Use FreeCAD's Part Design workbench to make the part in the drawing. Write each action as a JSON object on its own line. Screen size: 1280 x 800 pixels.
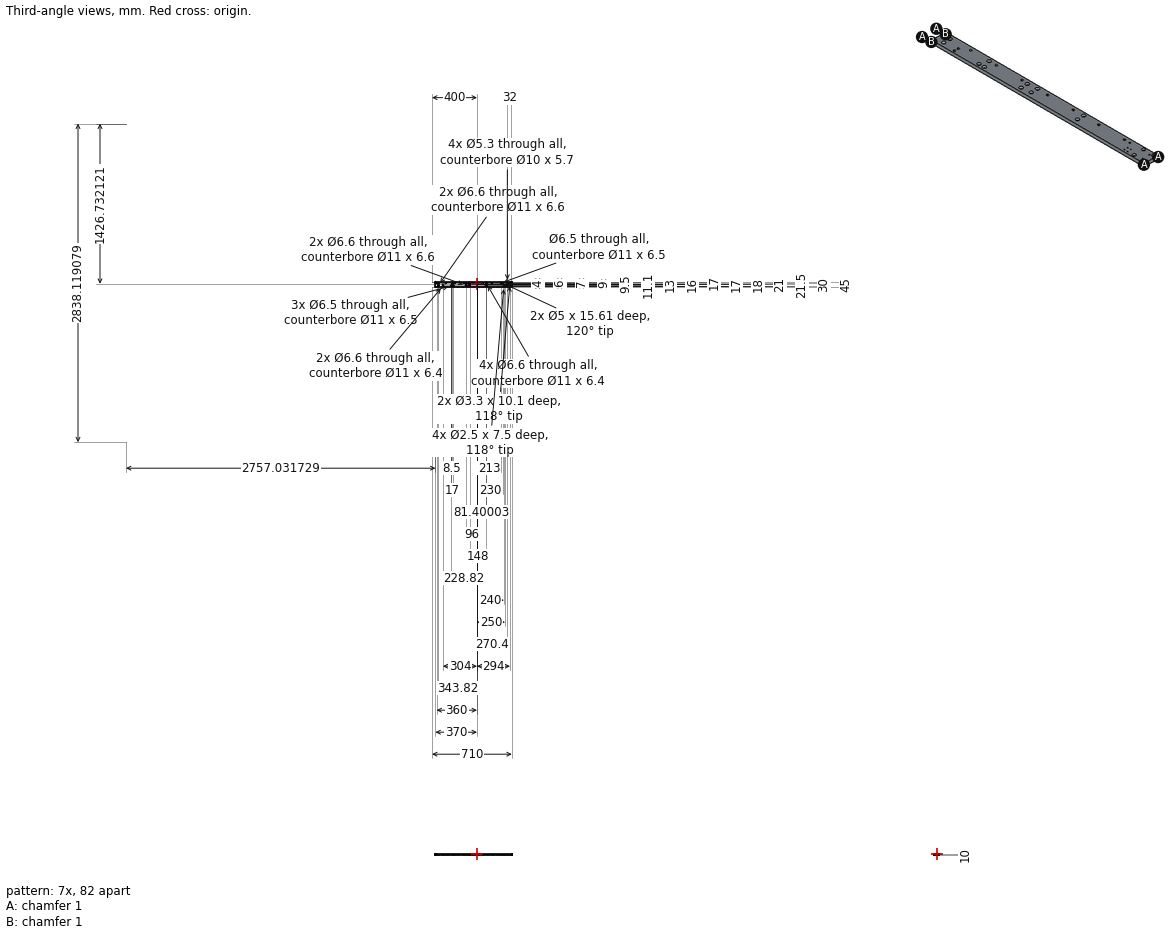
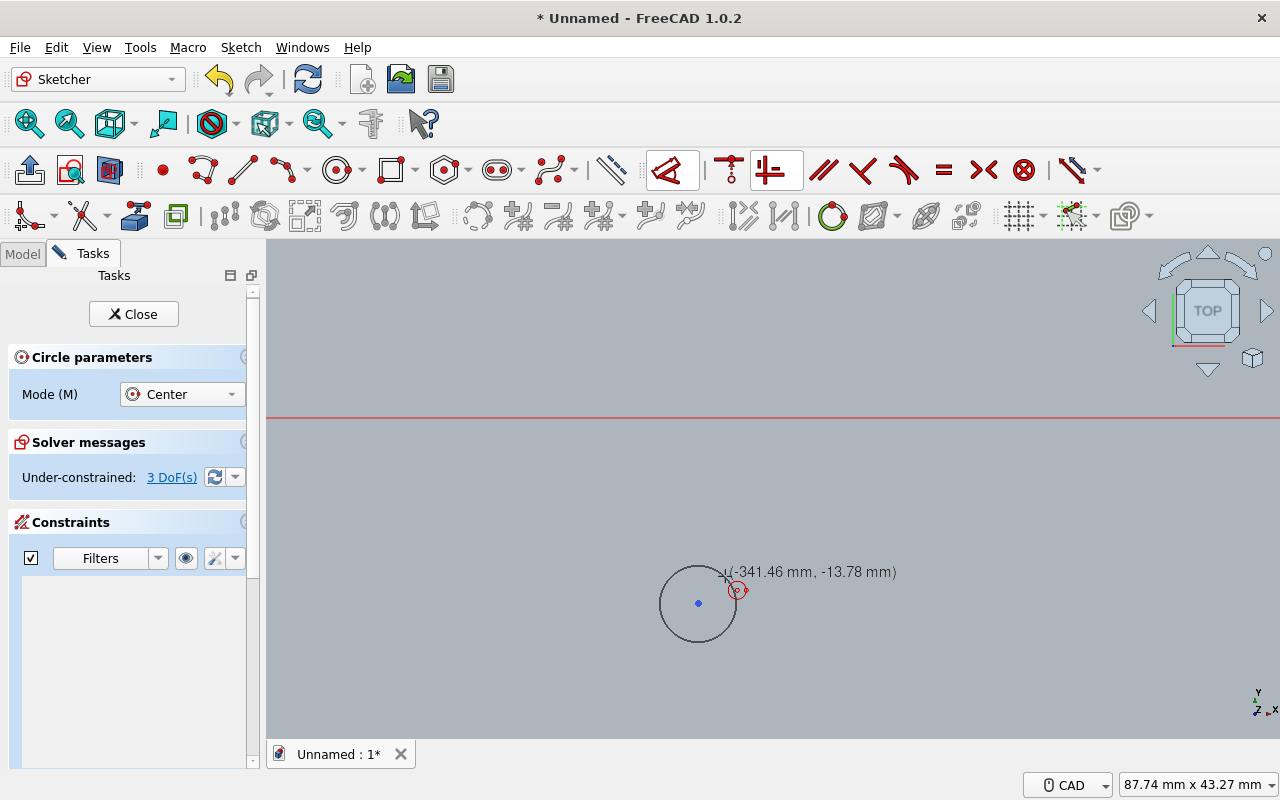
{"action": "left_click", "coordinate": [698, 371]}
{"action": "left_click", "coordinate": [725, 345]}
{"action": "key", "text": "Escape"}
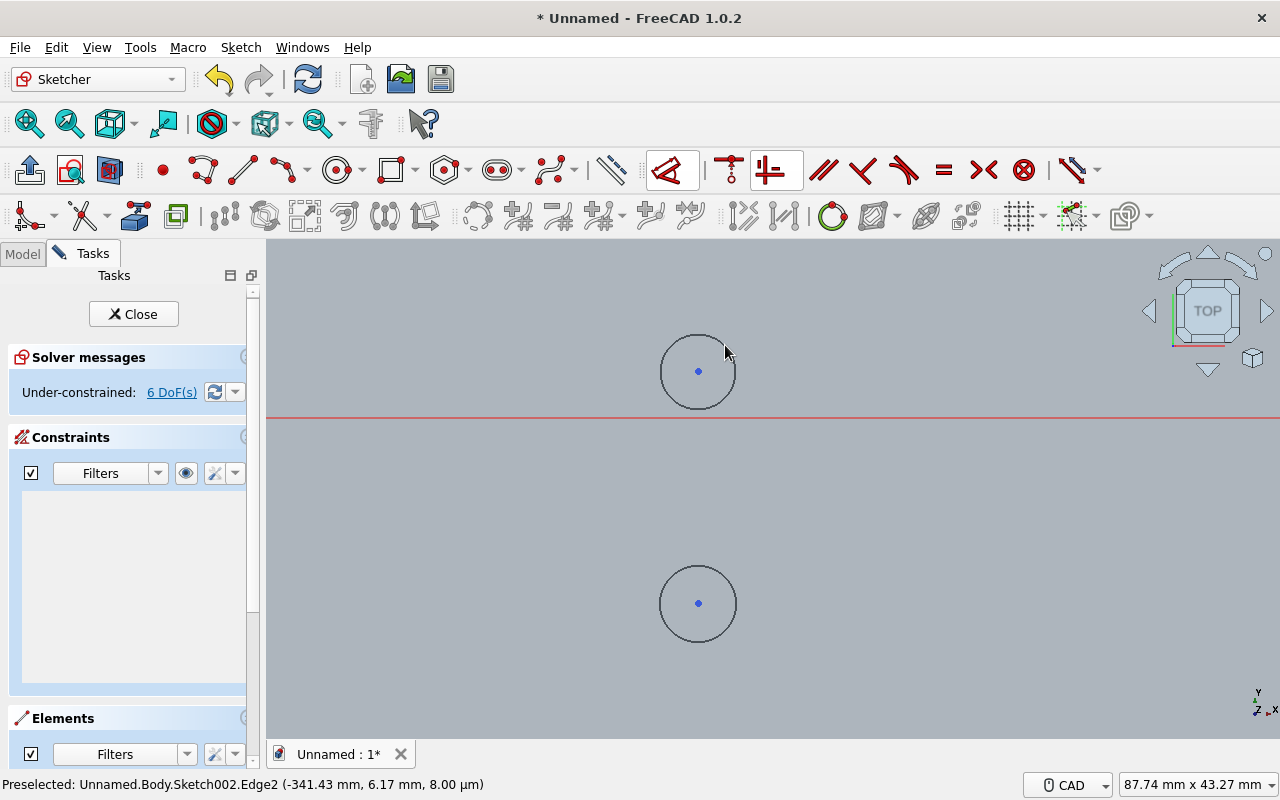
{"action": "left_click", "coordinate": [725, 577]}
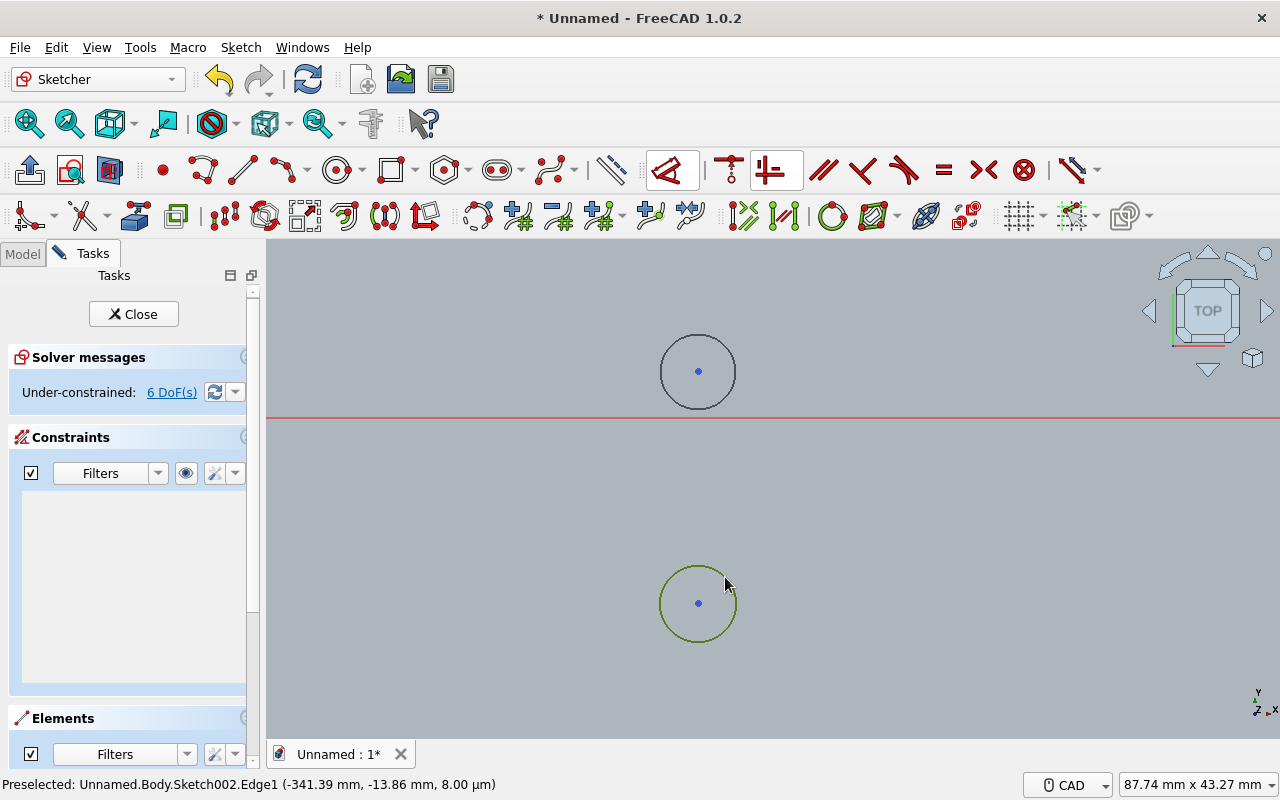
{"action": "left_click", "coordinate": [724, 345]}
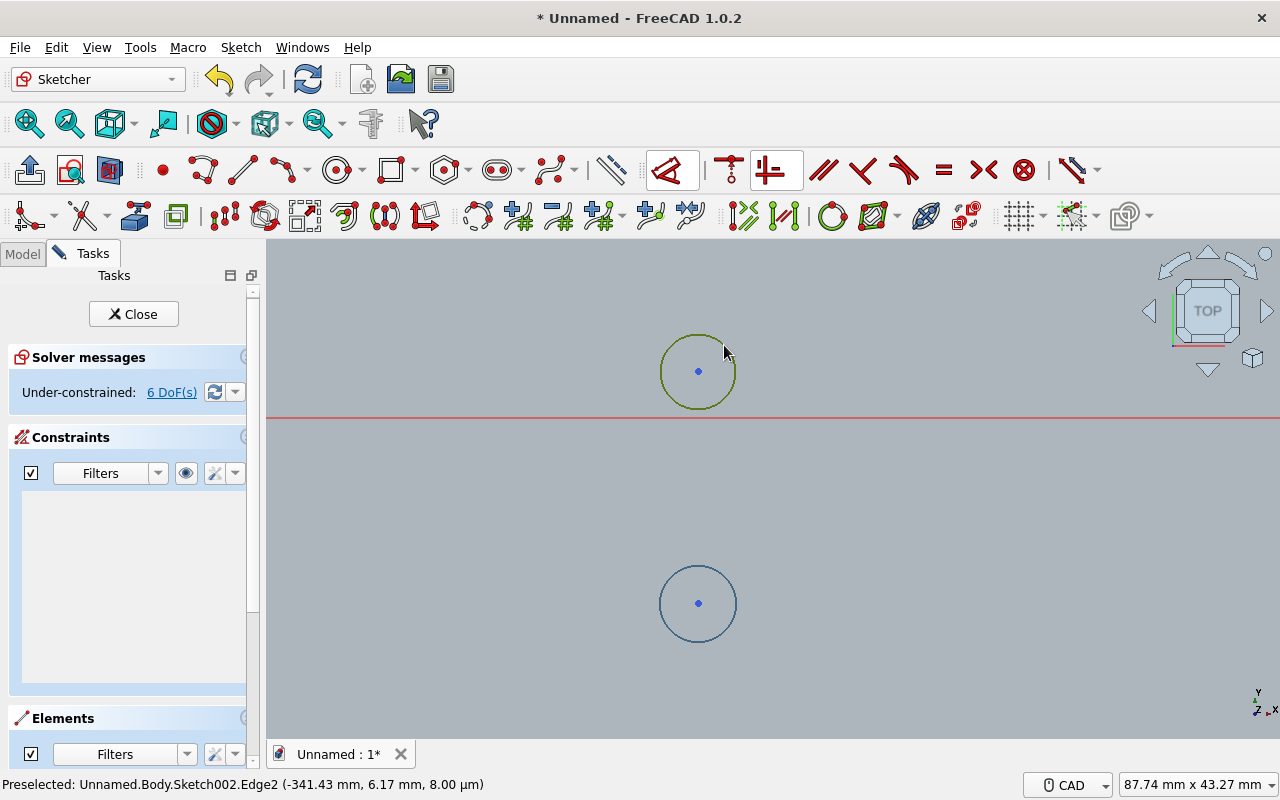
{"action": "left_click", "coordinate": [944, 170]}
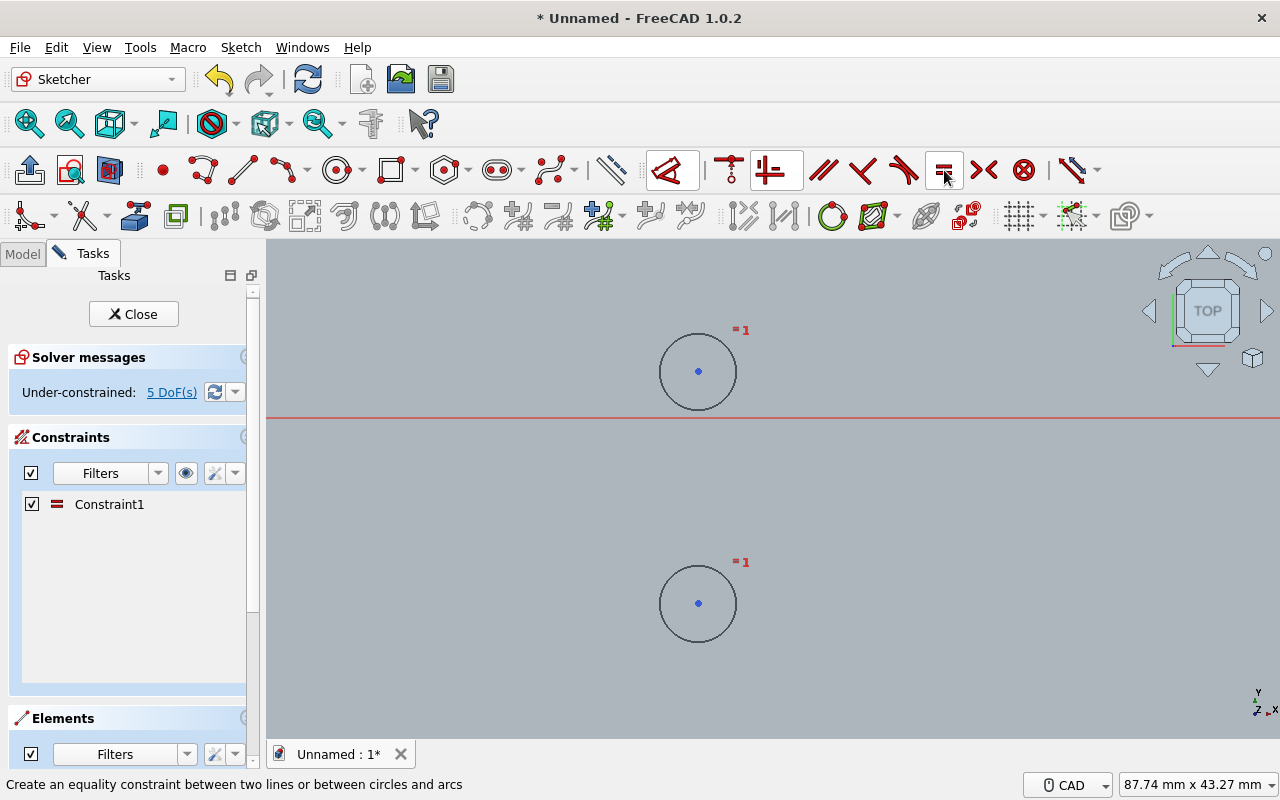
{"action": "left_click", "coordinate": [698, 604]}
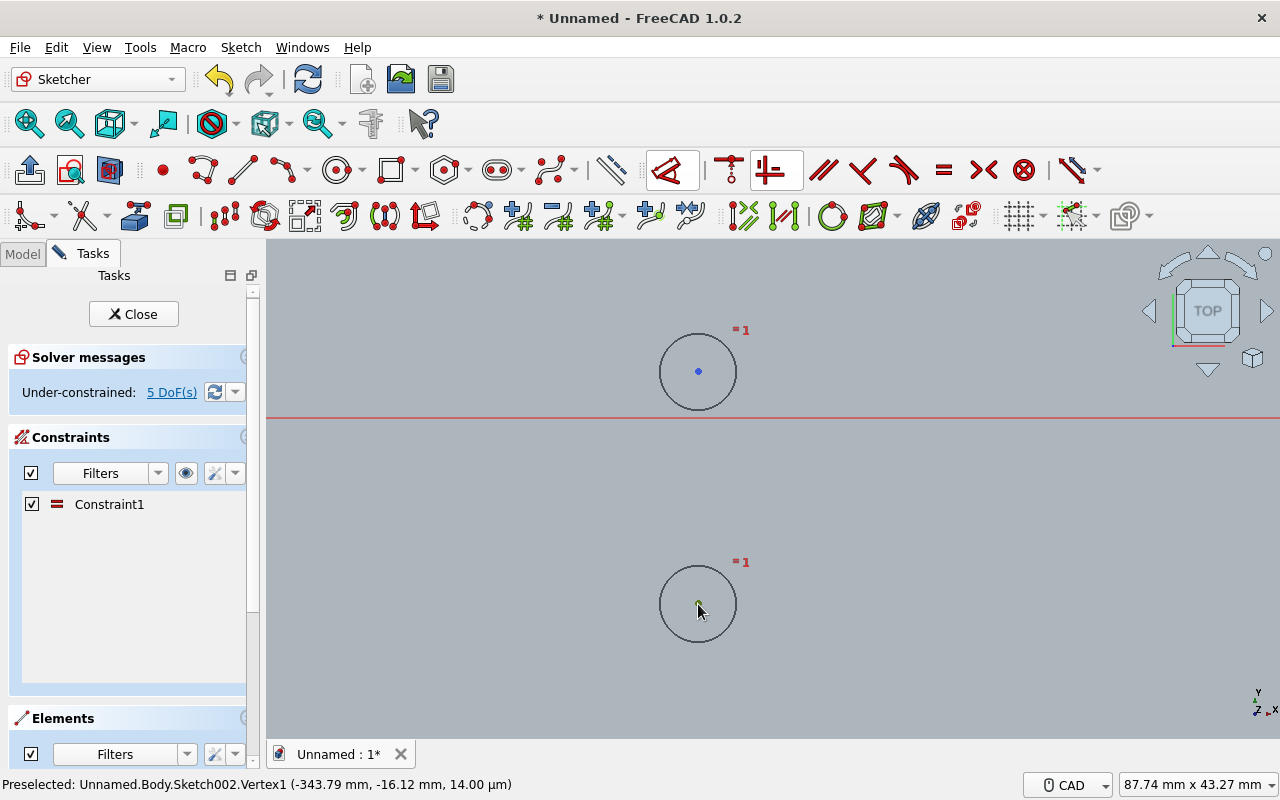
{"action": "left_click", "coordinate": [698, 372]}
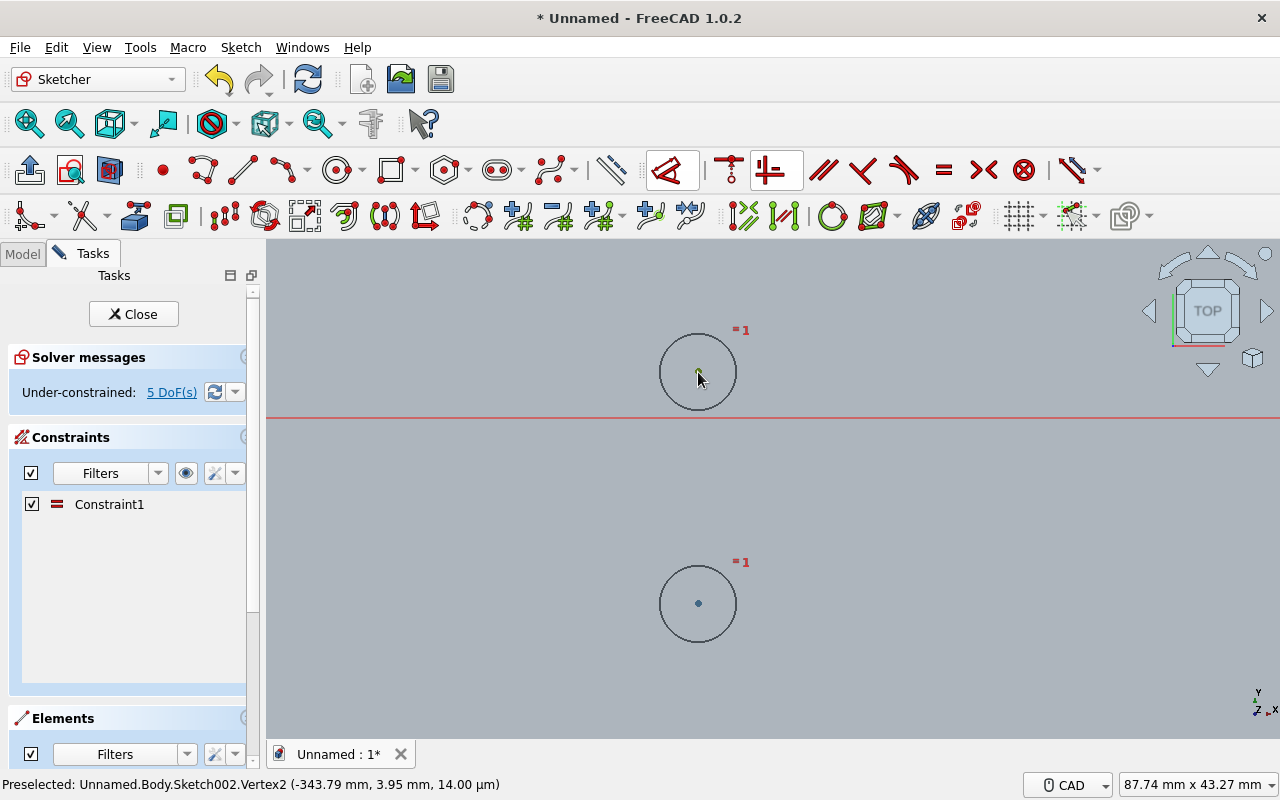
{"action": "key", "text": "v"}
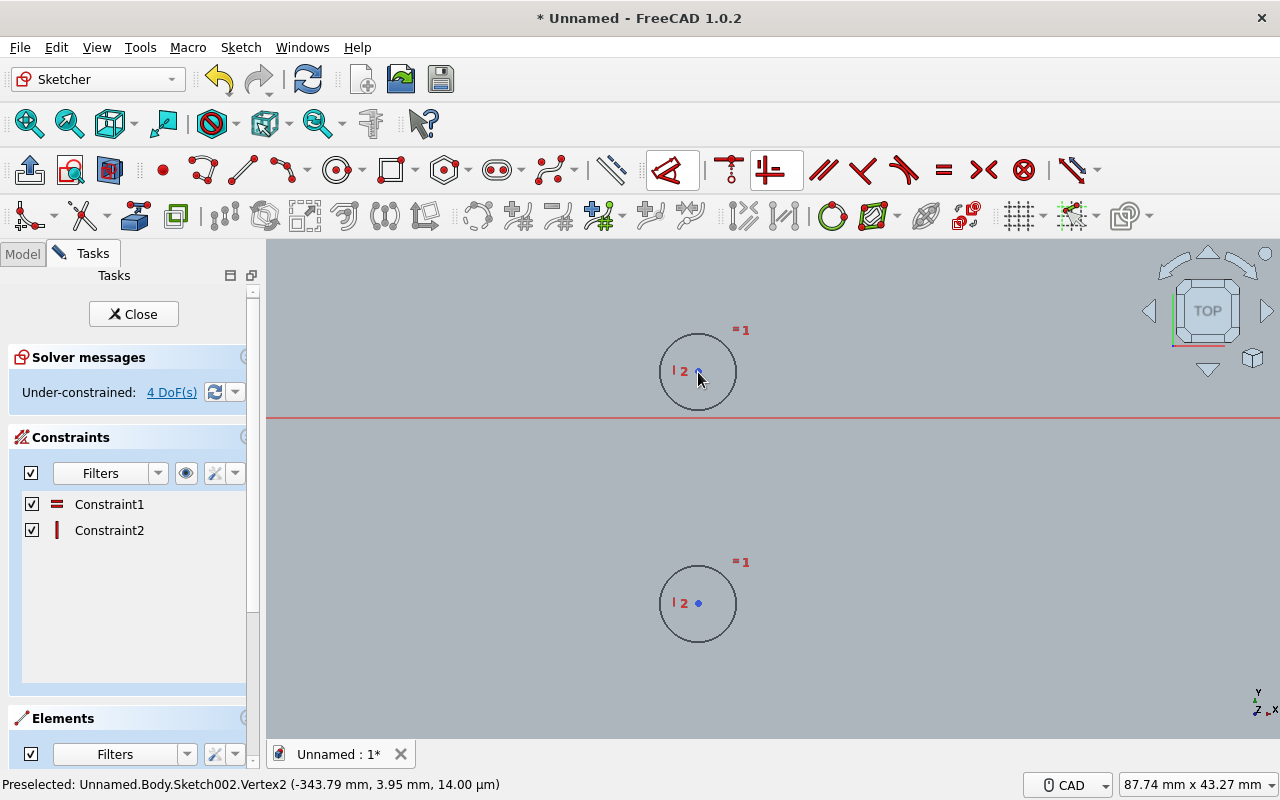
{"action": "left_click", "coordinate": [725, 577]}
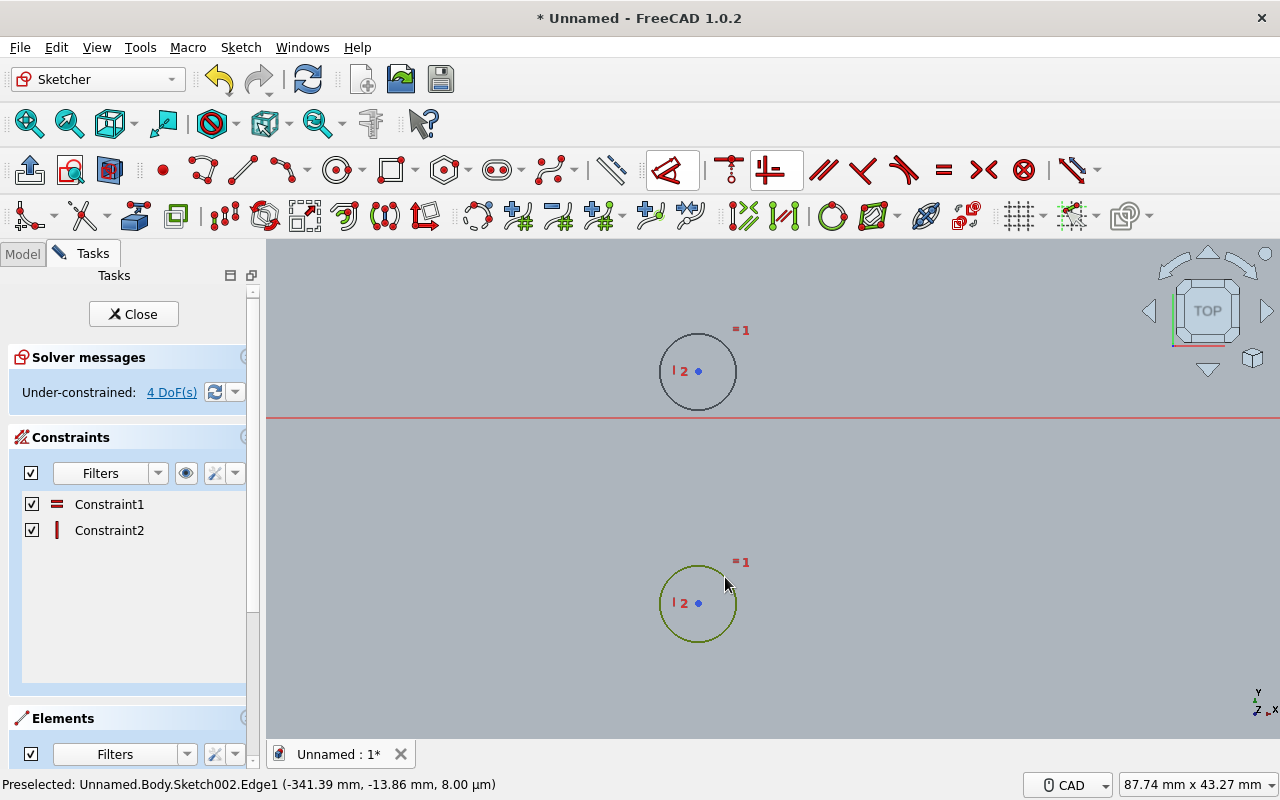
{"action": "left_click", "coordinate": [694, 170]}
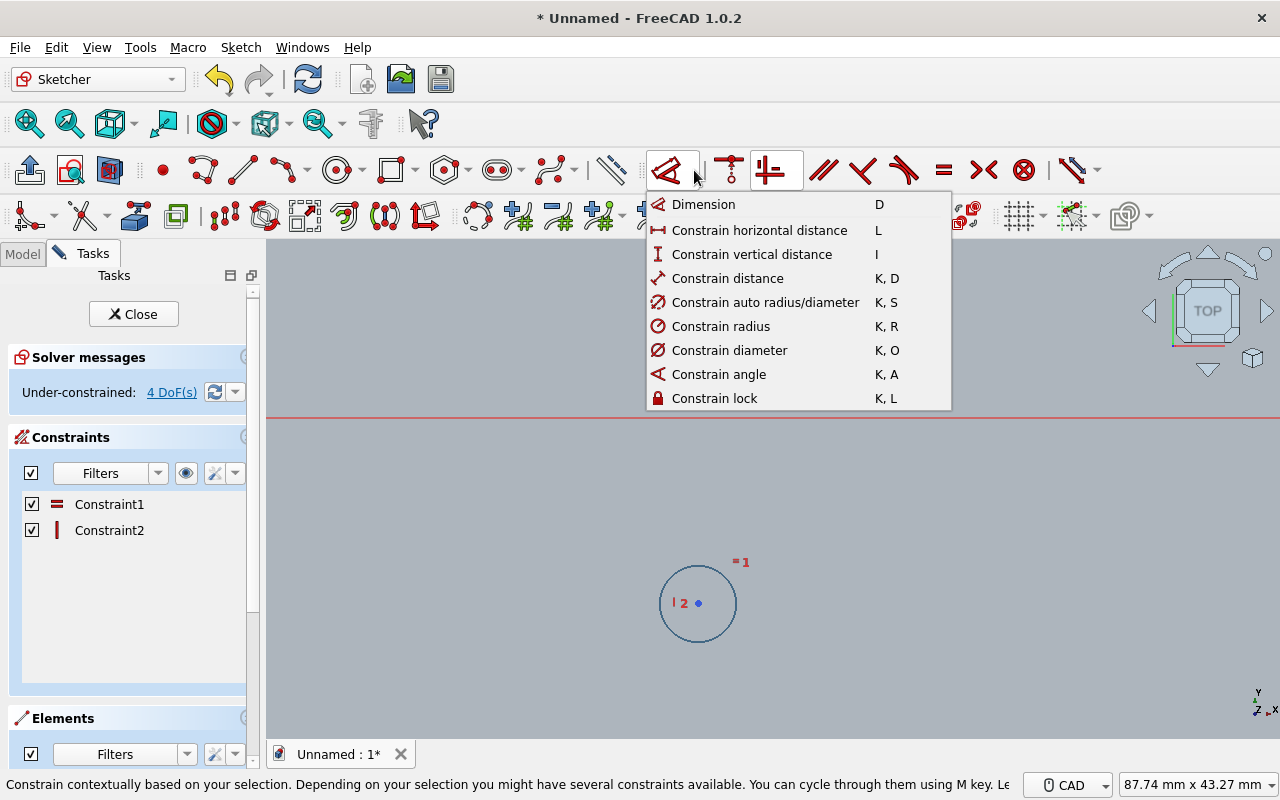
{"action": "left_click", "coordinate": [799, 350]}